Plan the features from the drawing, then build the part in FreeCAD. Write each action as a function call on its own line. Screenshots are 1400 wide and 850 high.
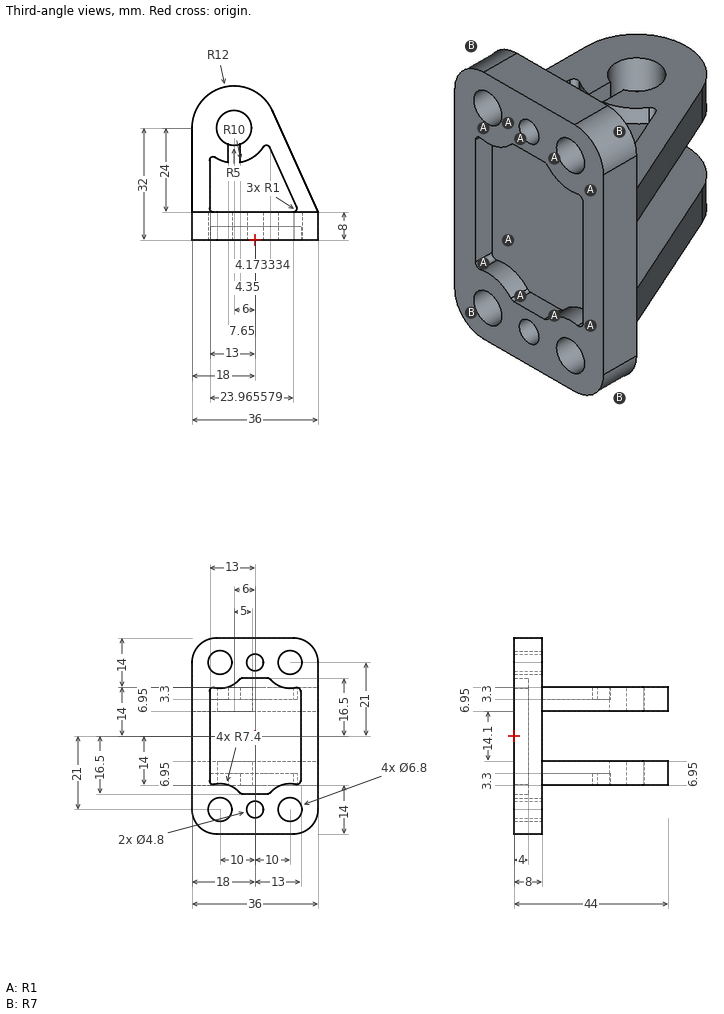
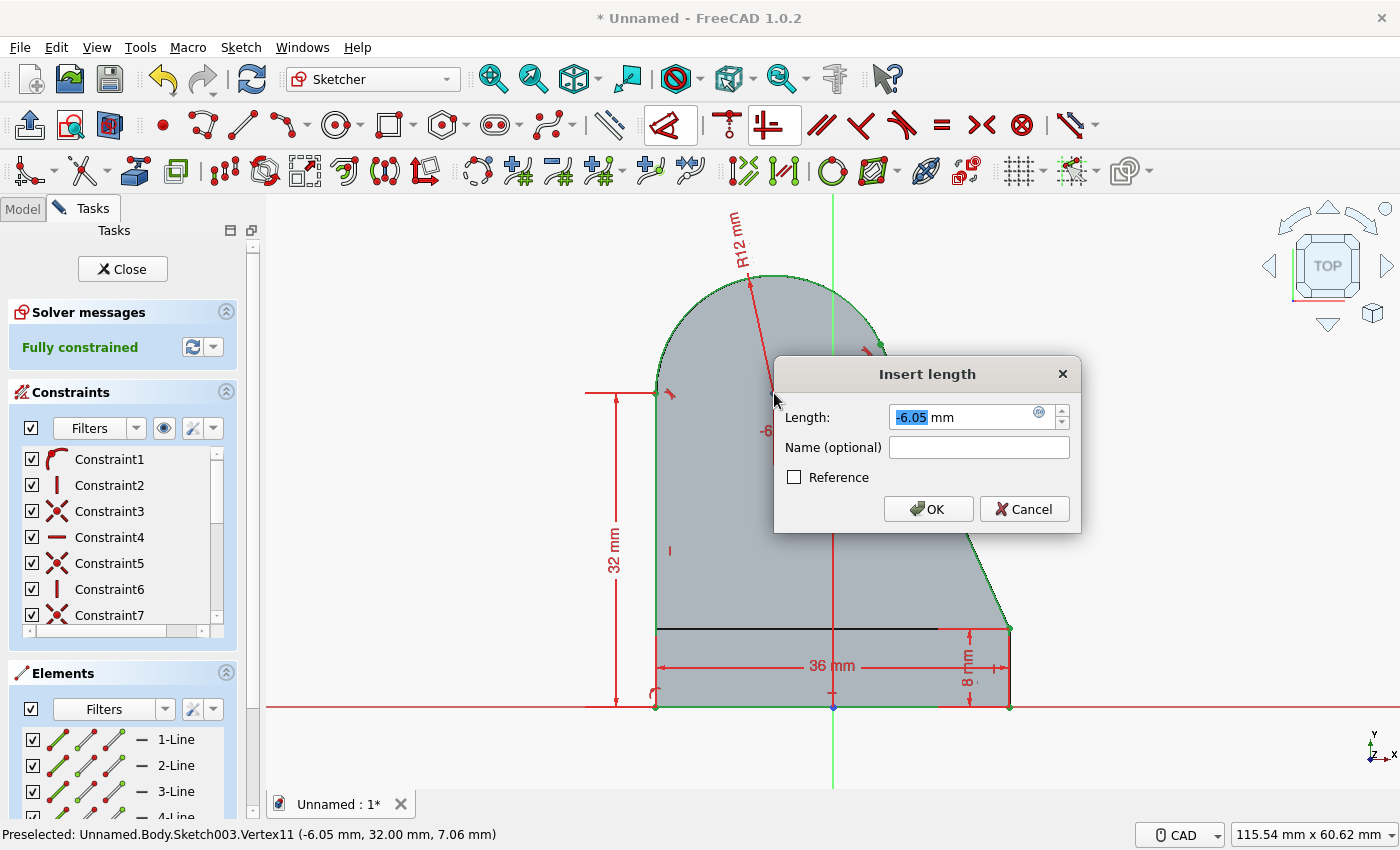
text(-6)
key(Return)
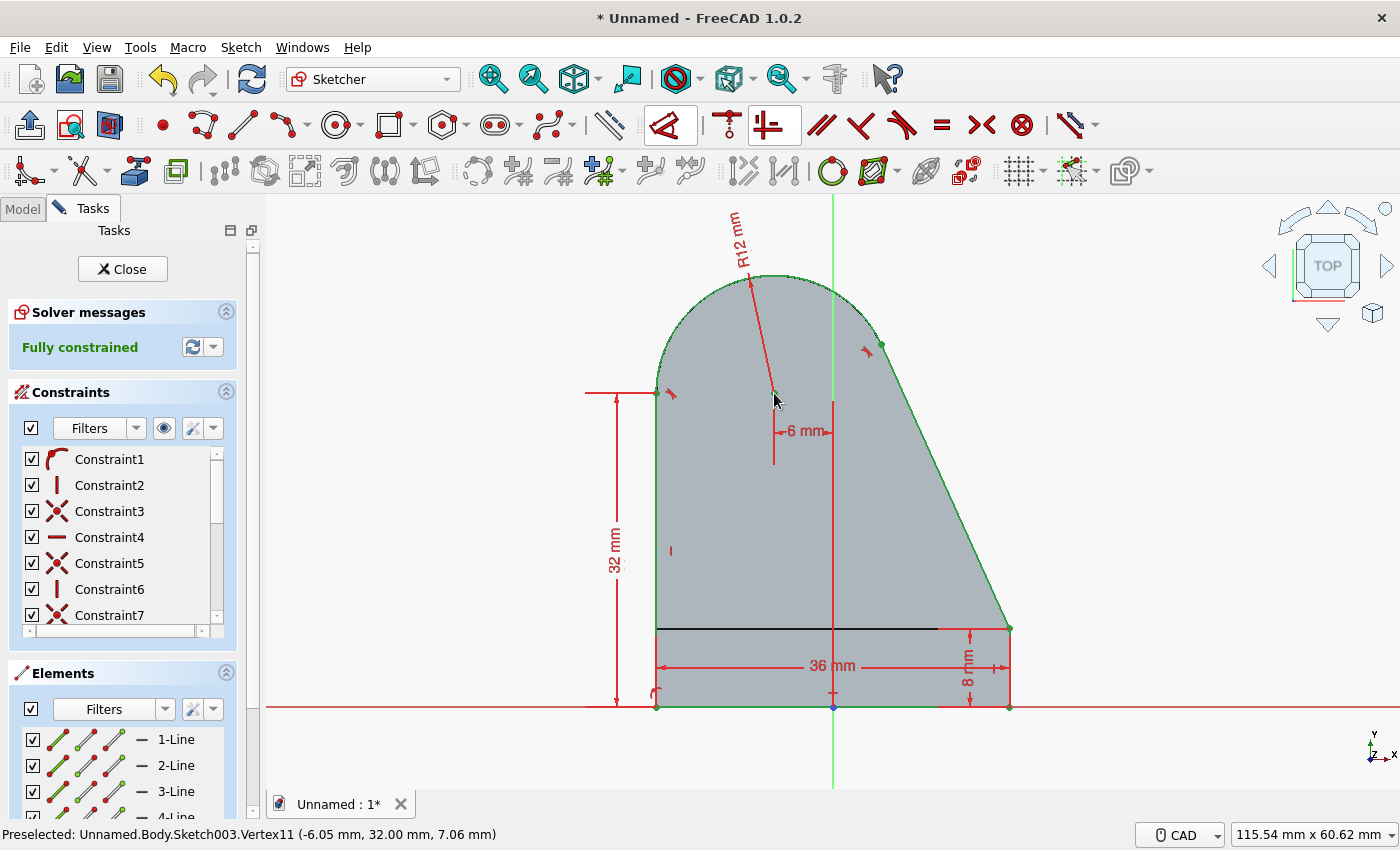
click(123, 269)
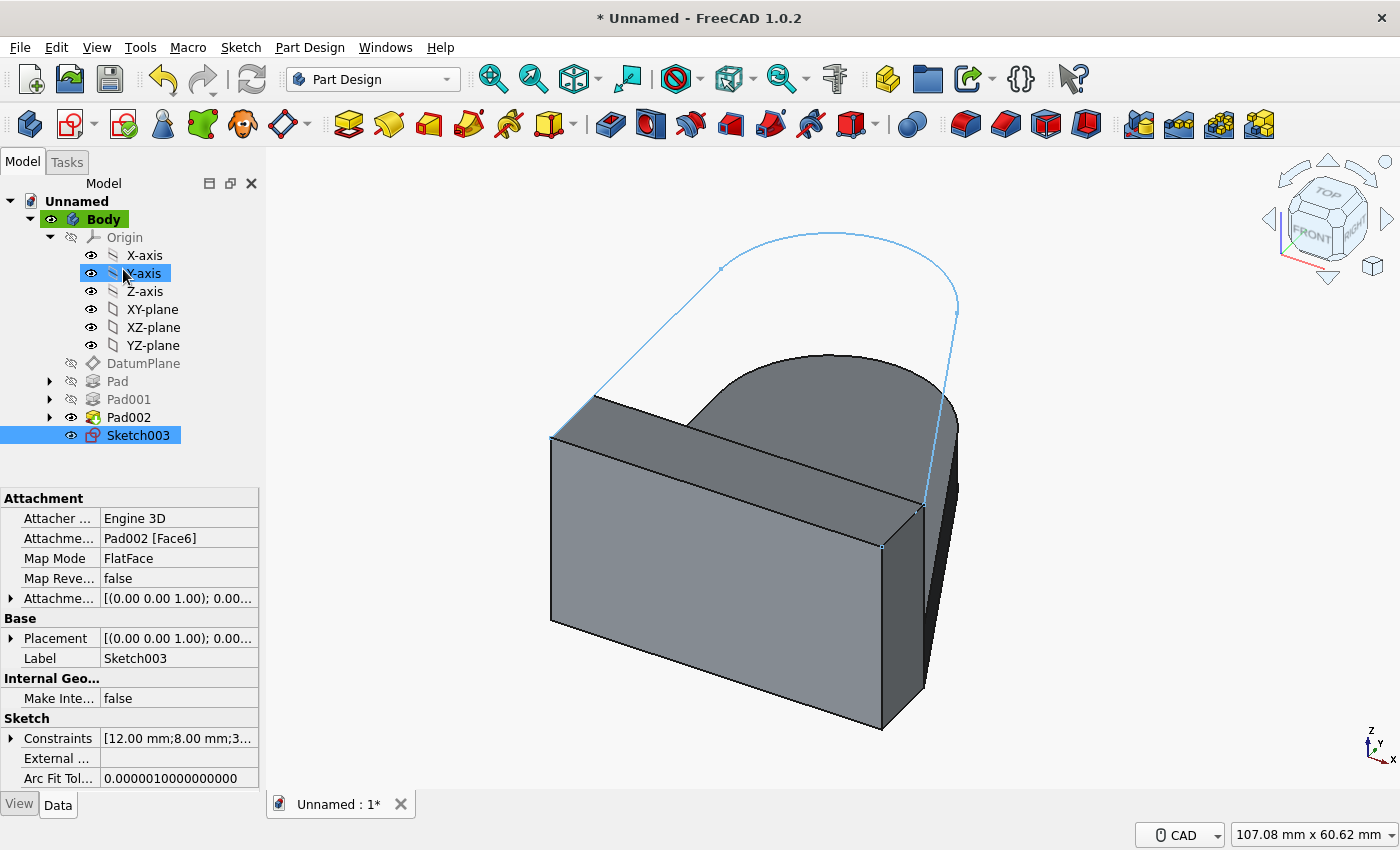
click(350, 124)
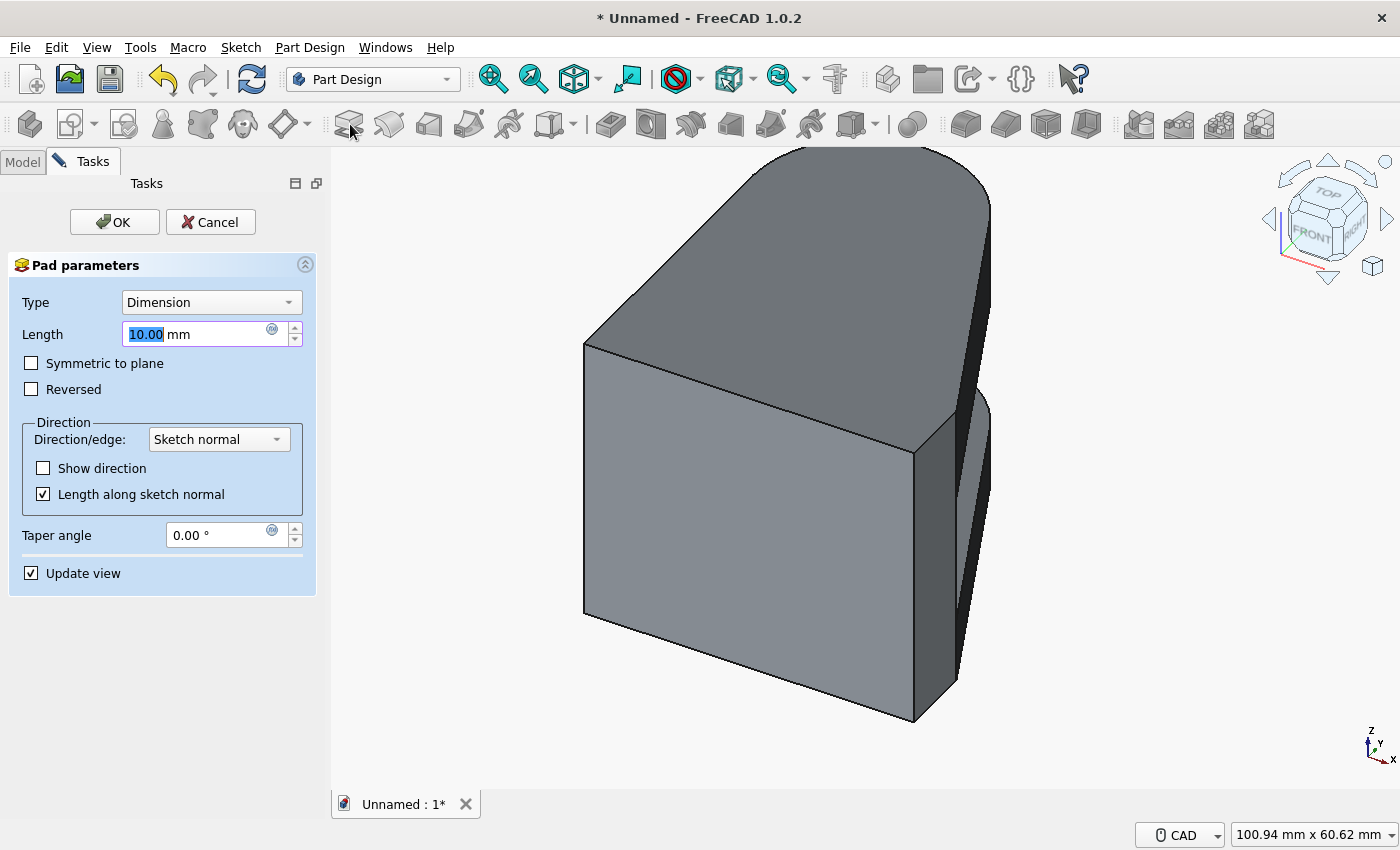
text(6.95)
key(Tab)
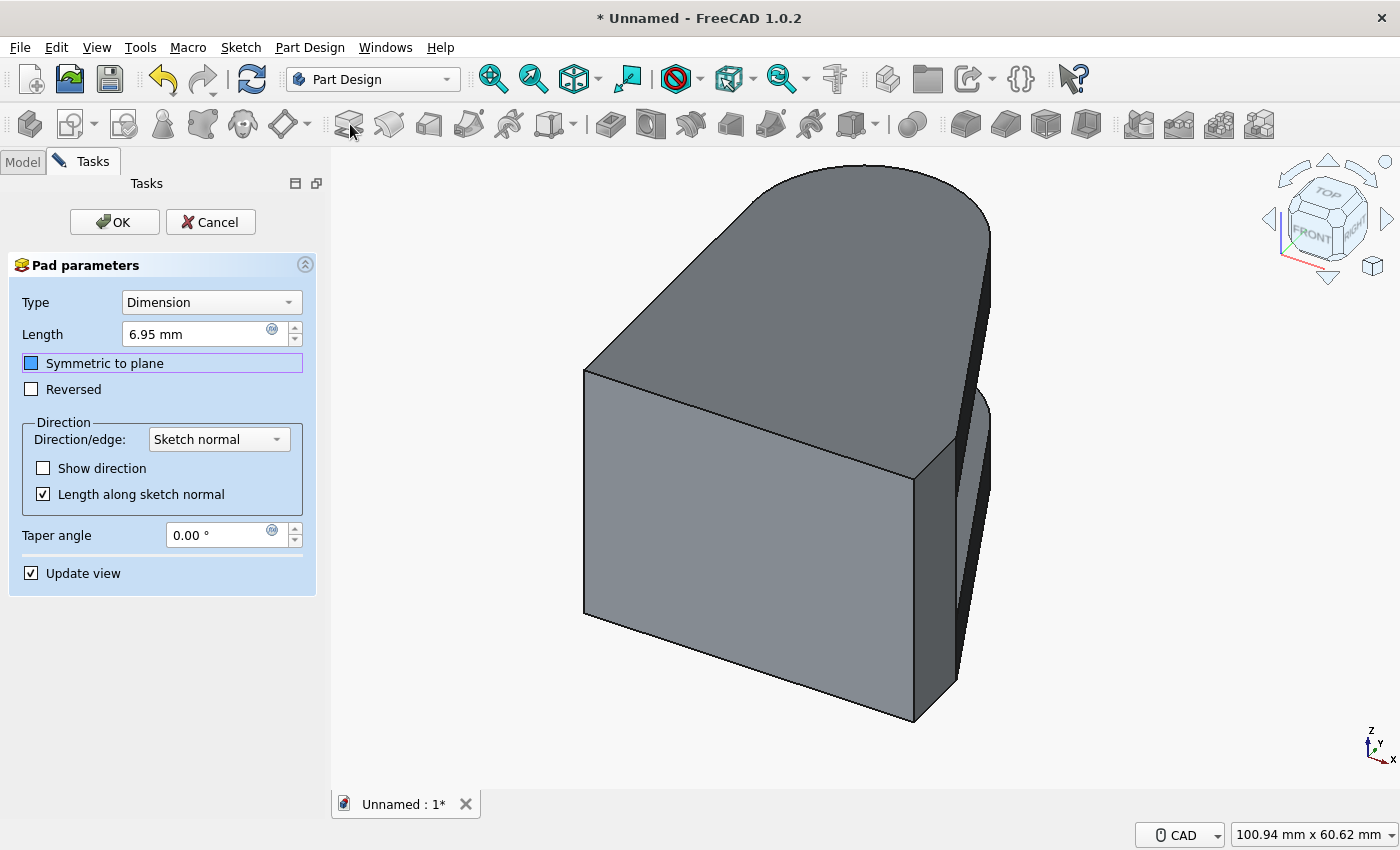
click(115, 222)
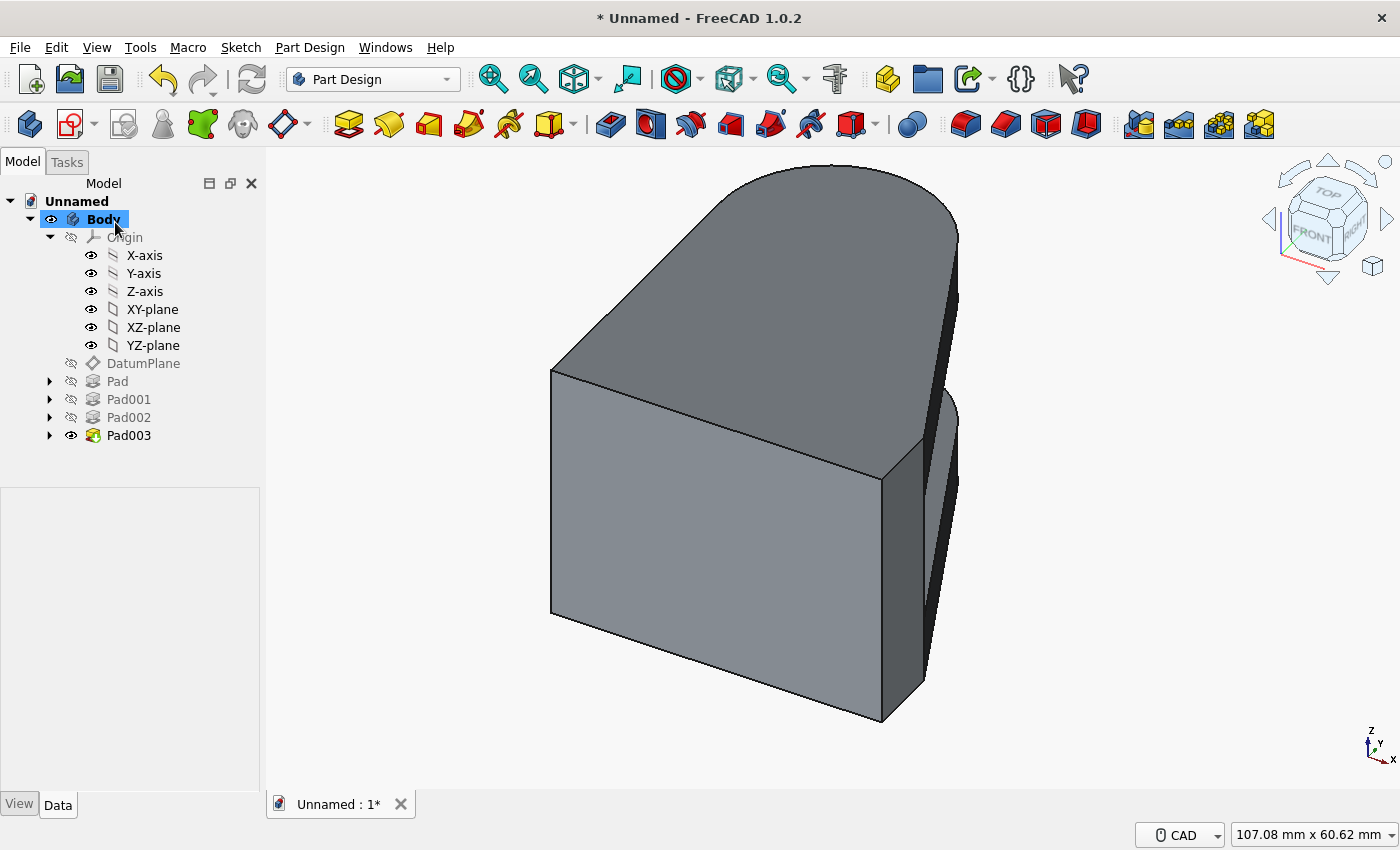
click(494, 80)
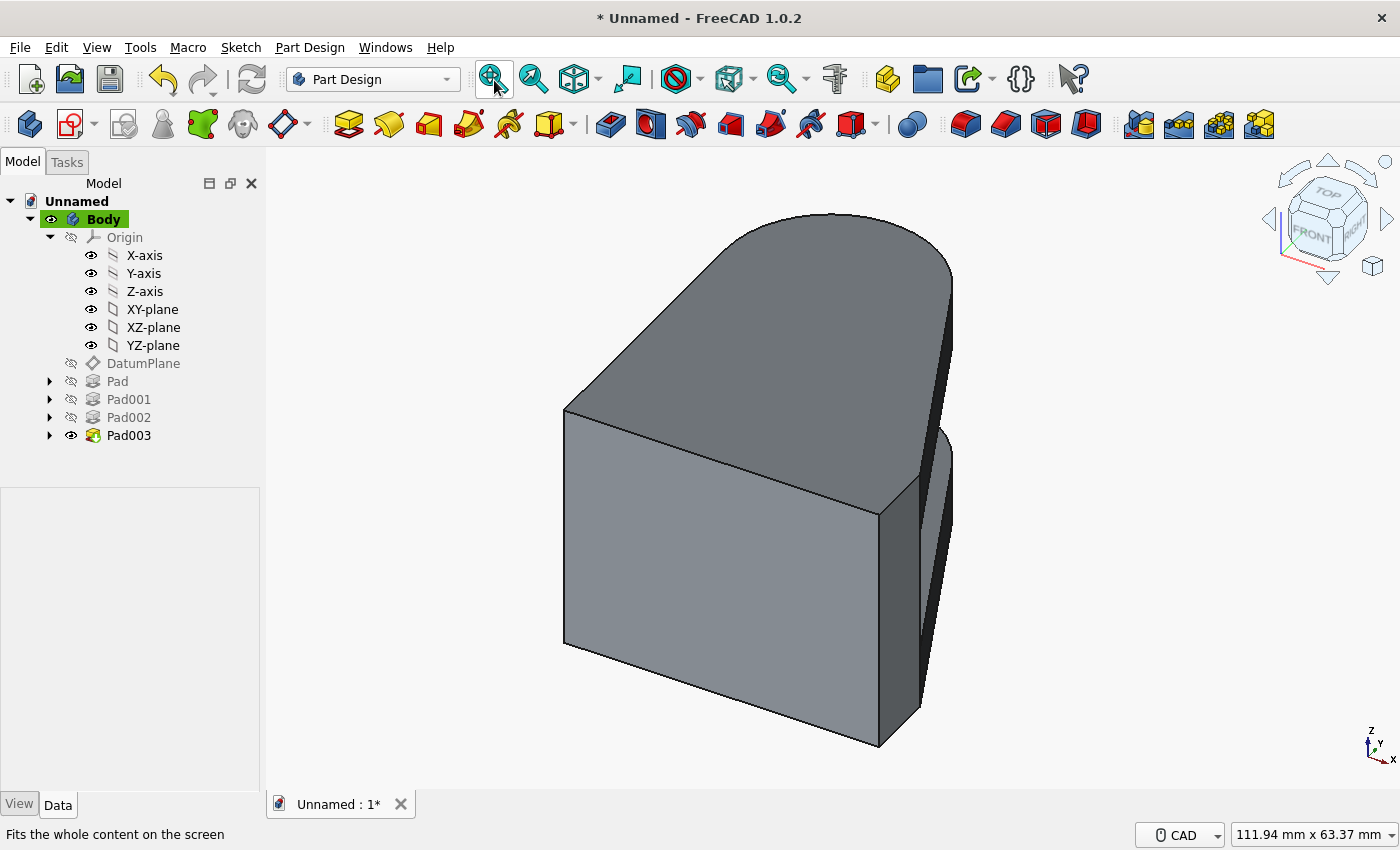
click(801, 382)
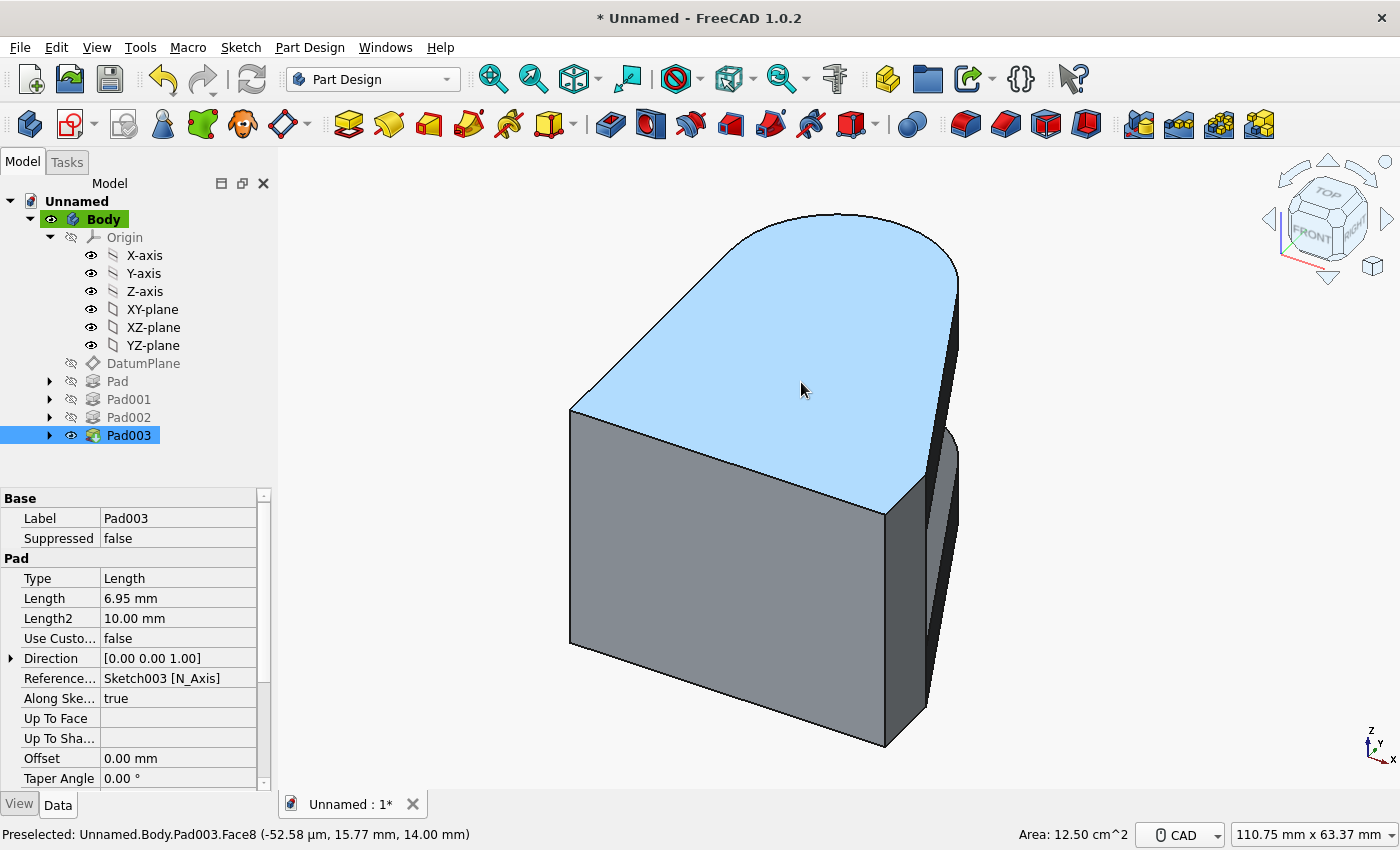
click(70, 124)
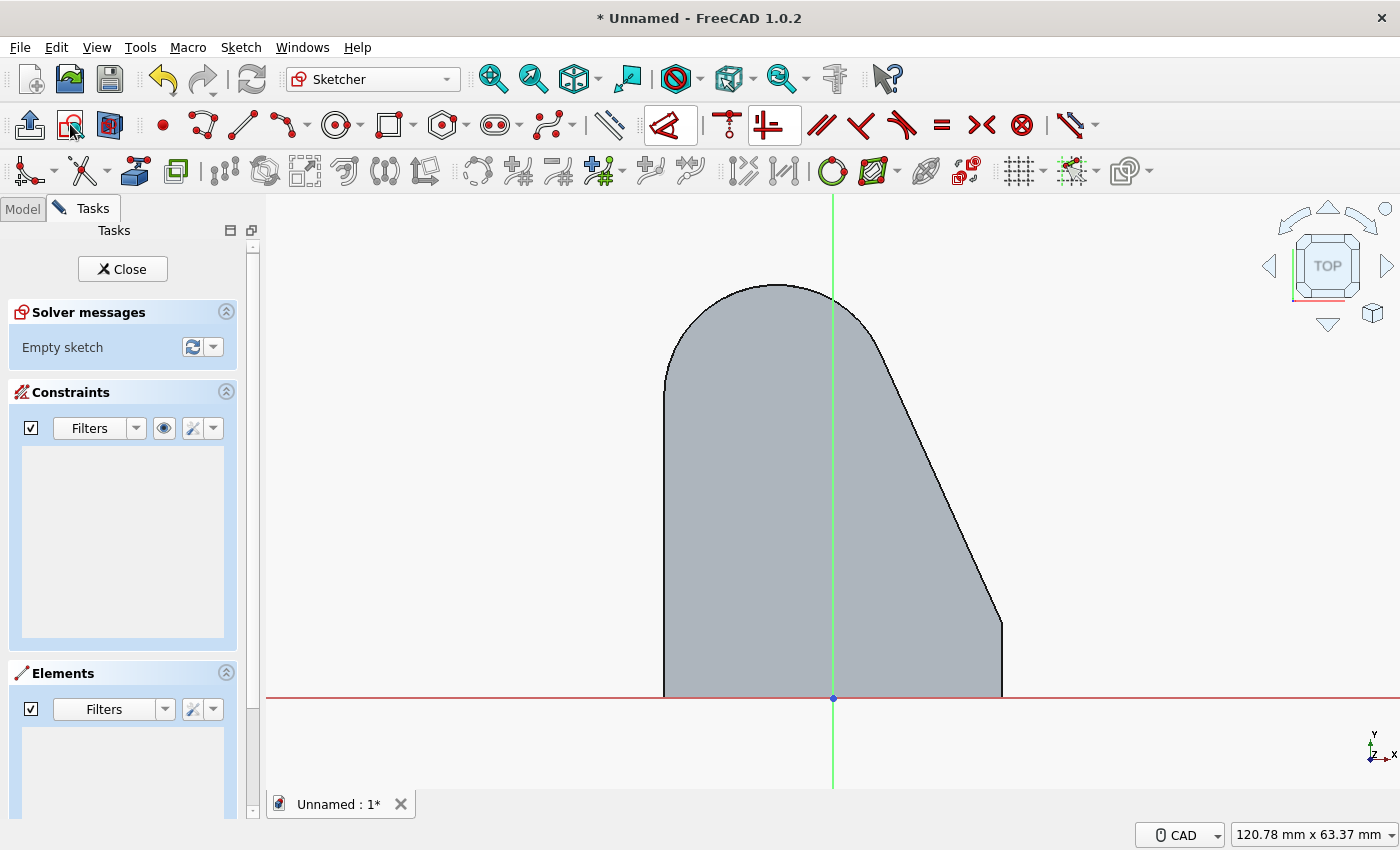
scroll(916, 761, up, 3)